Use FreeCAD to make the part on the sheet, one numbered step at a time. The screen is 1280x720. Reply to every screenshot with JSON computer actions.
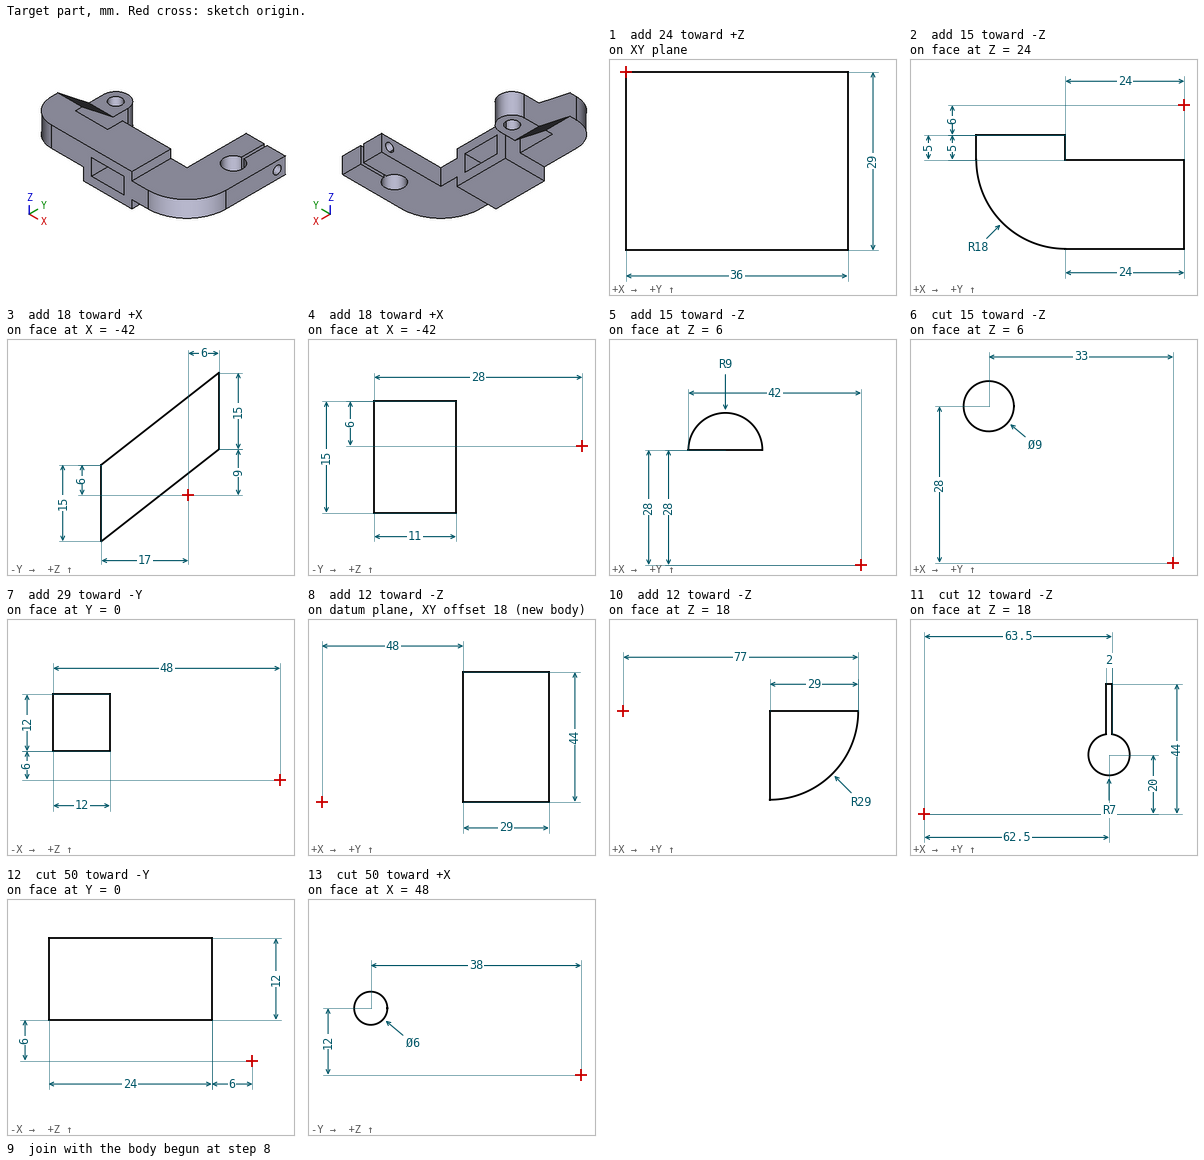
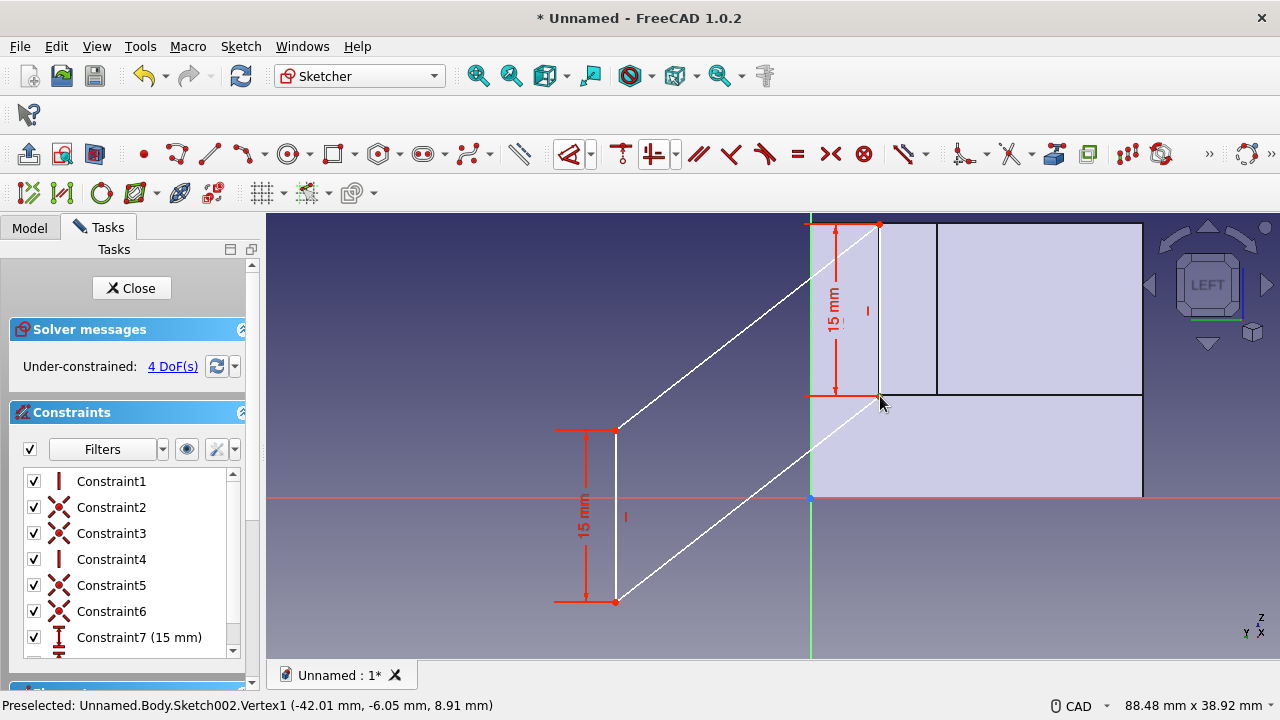
{"action": "key", "text": "l"}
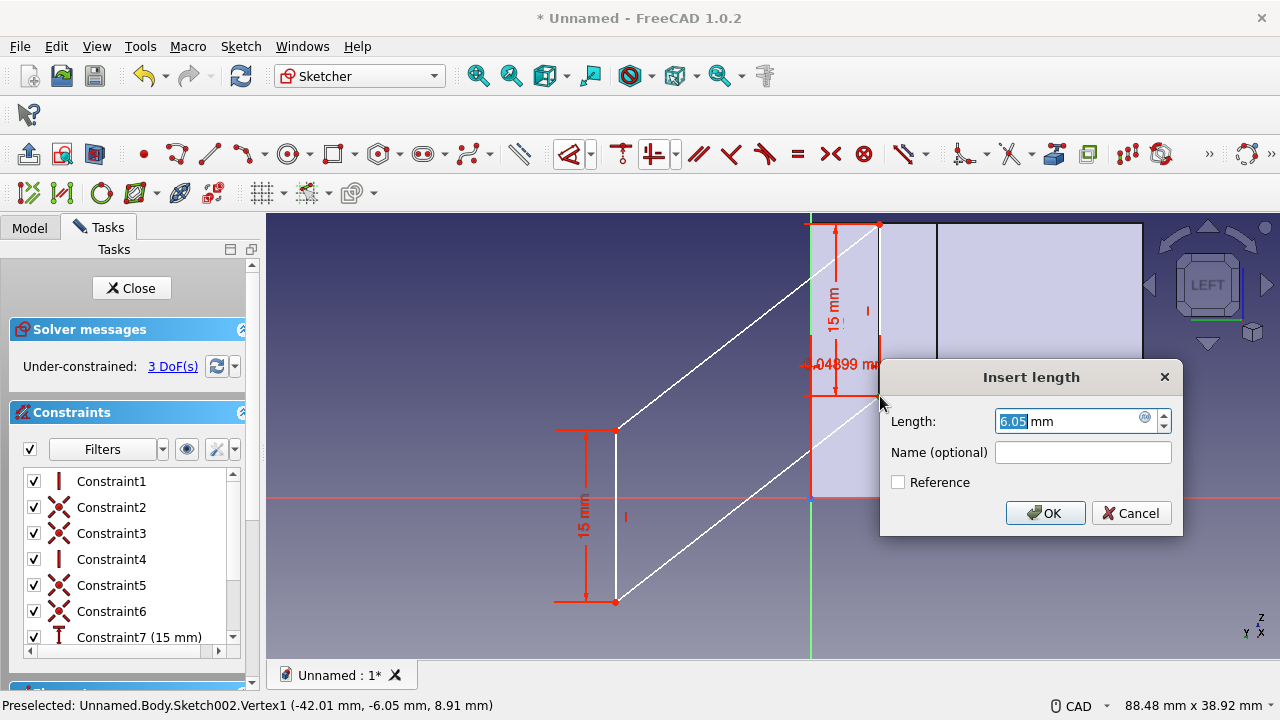
{"action": "type", "text": "6"}
{"action": "key", "text": "Return"}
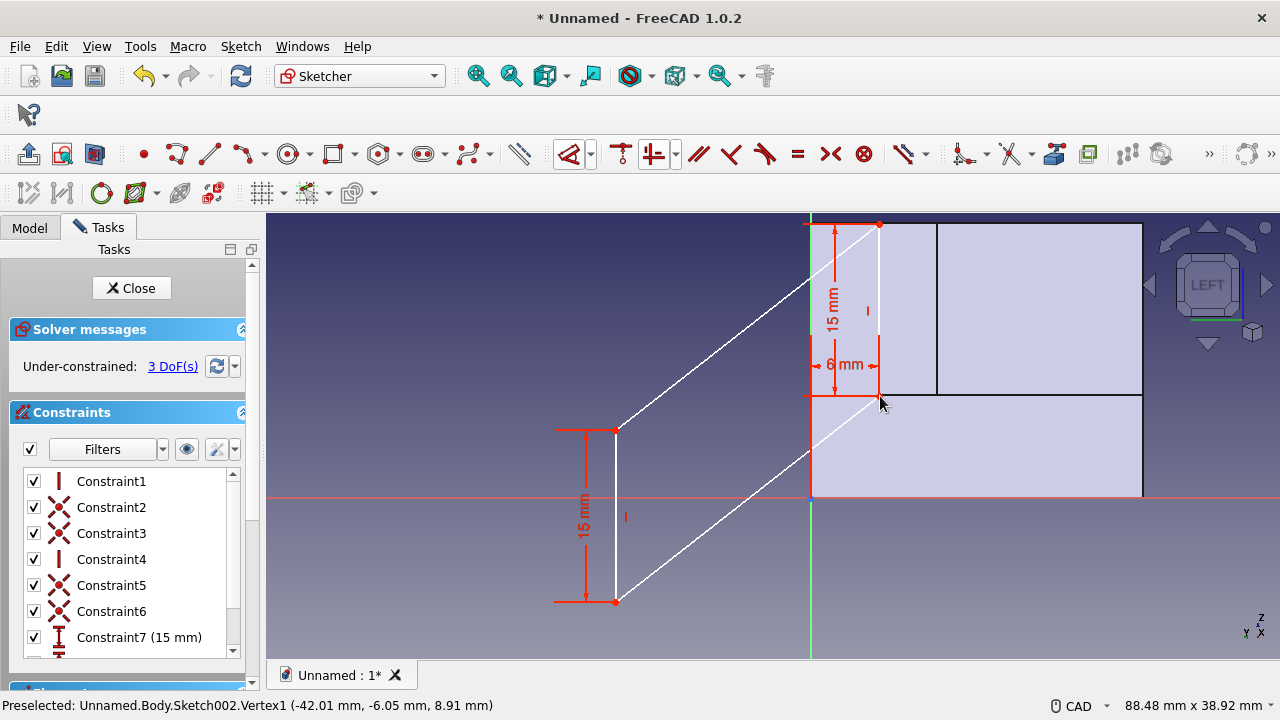
{"action": "left_click", "coordinate": [879, 396]}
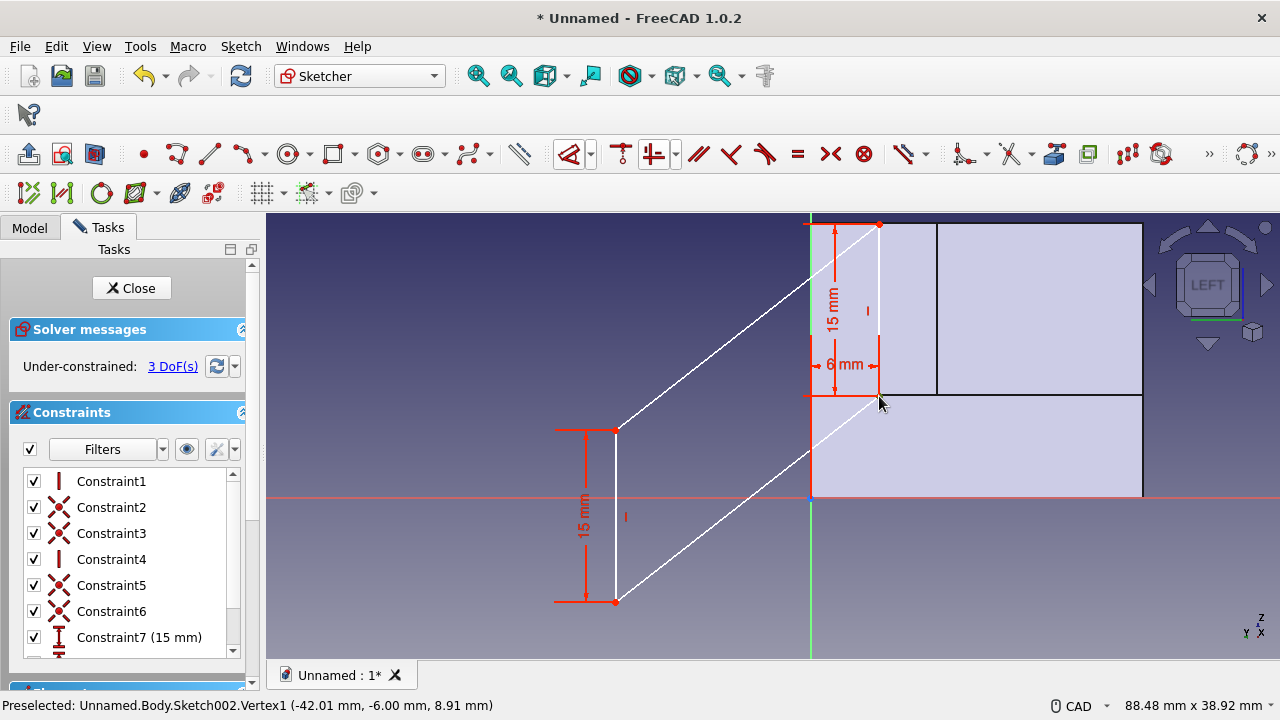
{"action": "left_click", "coordinate": [590, 154]}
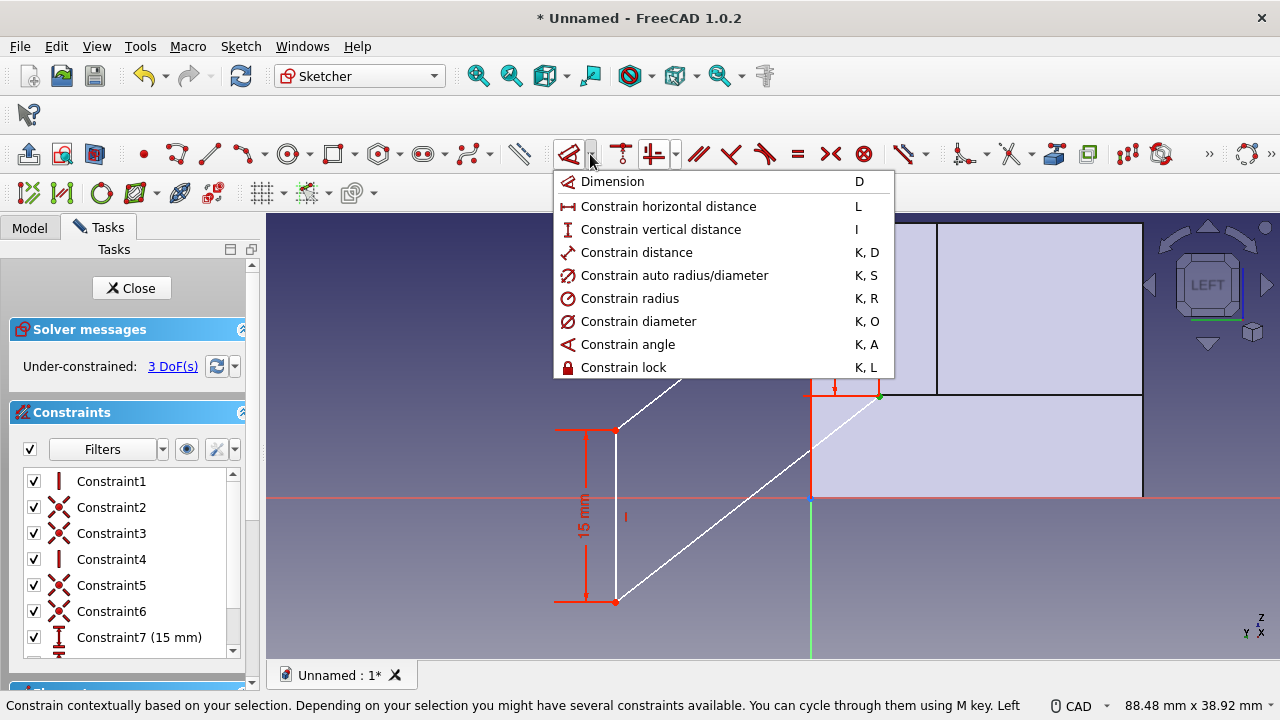
{"action": "left_click", "coordinate": [724, 230]}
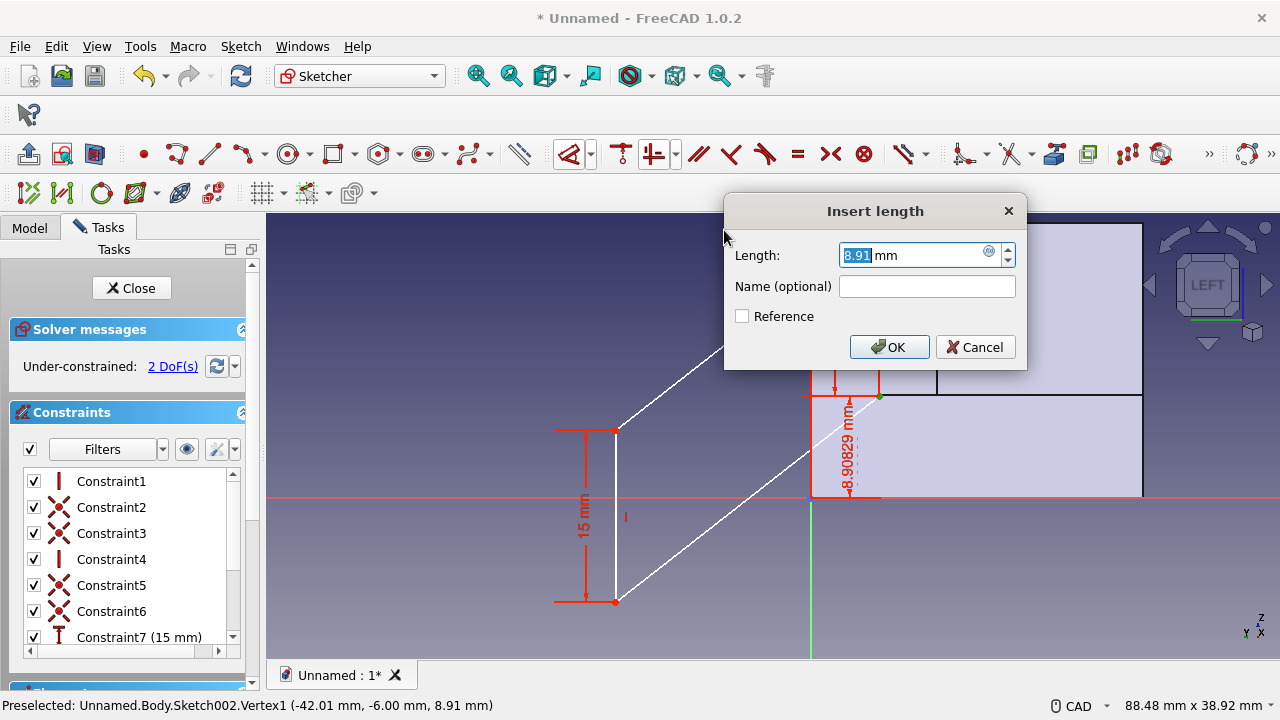
{"action": "type", "text": "9"}
{"action": "key", "text": "Return"}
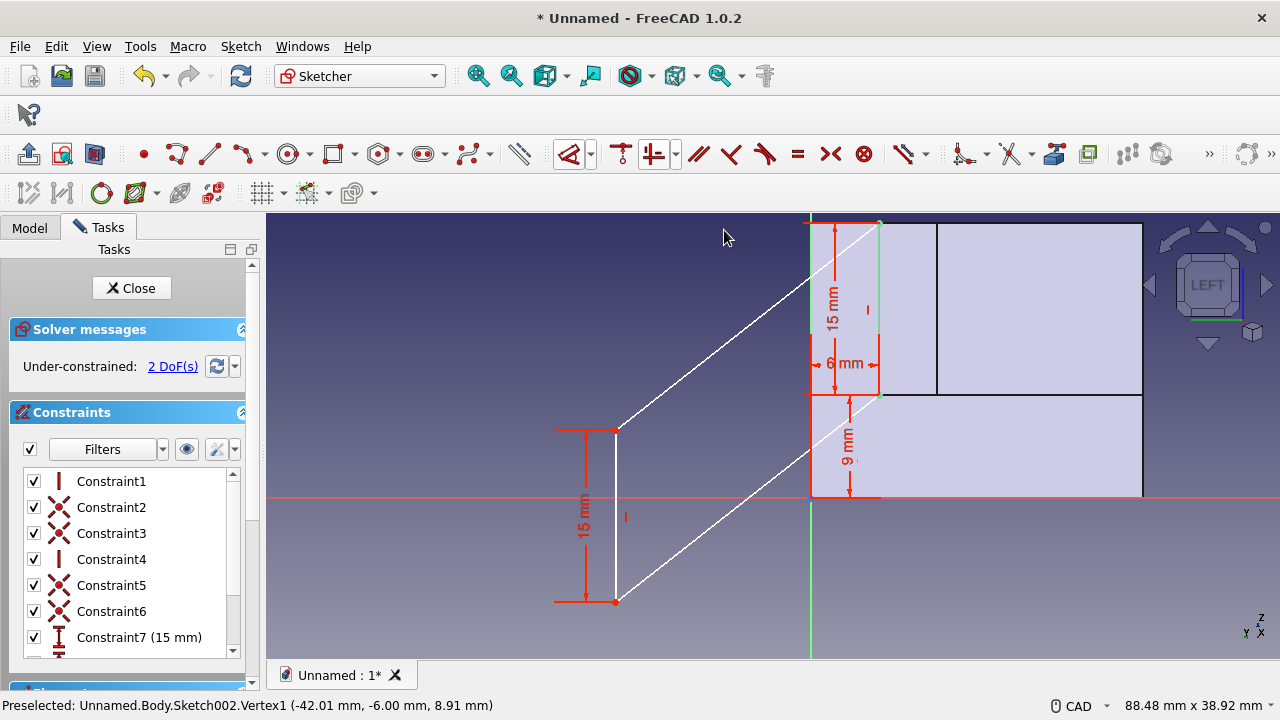
{"action": "left_click", "coordinate": [616, 430]}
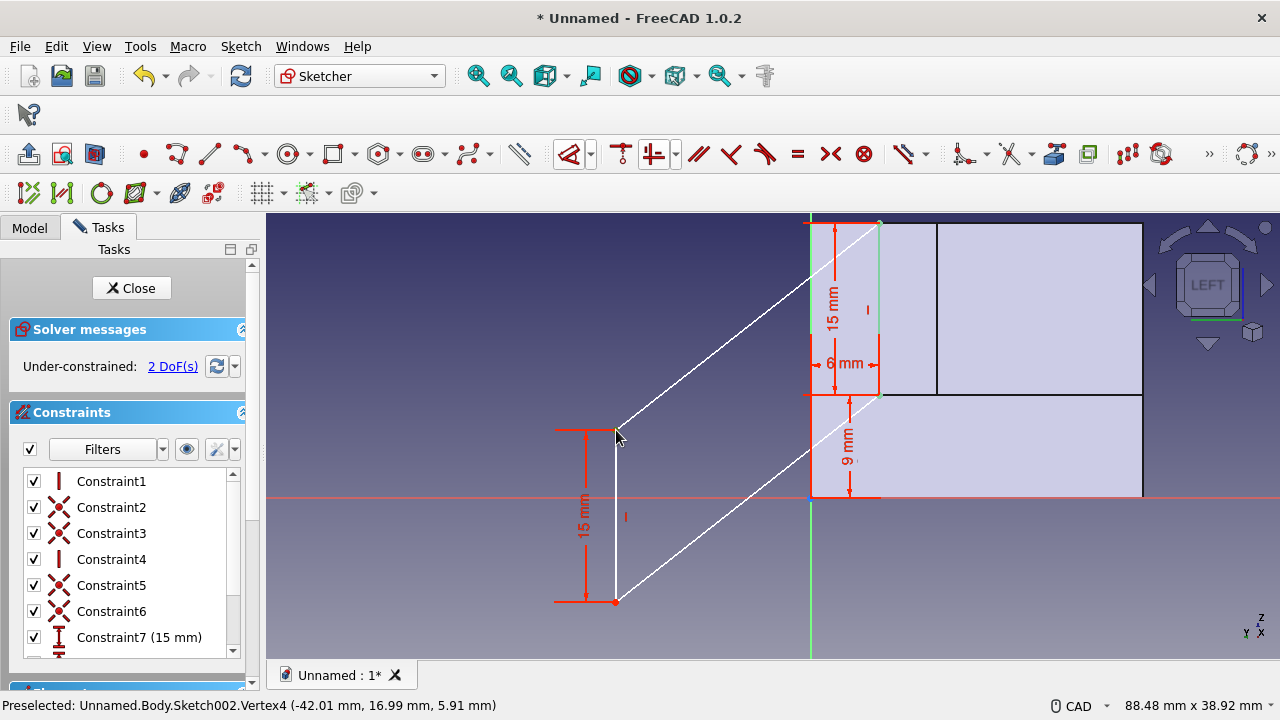
{"action": "left_click", "coordinate": [590, 154]}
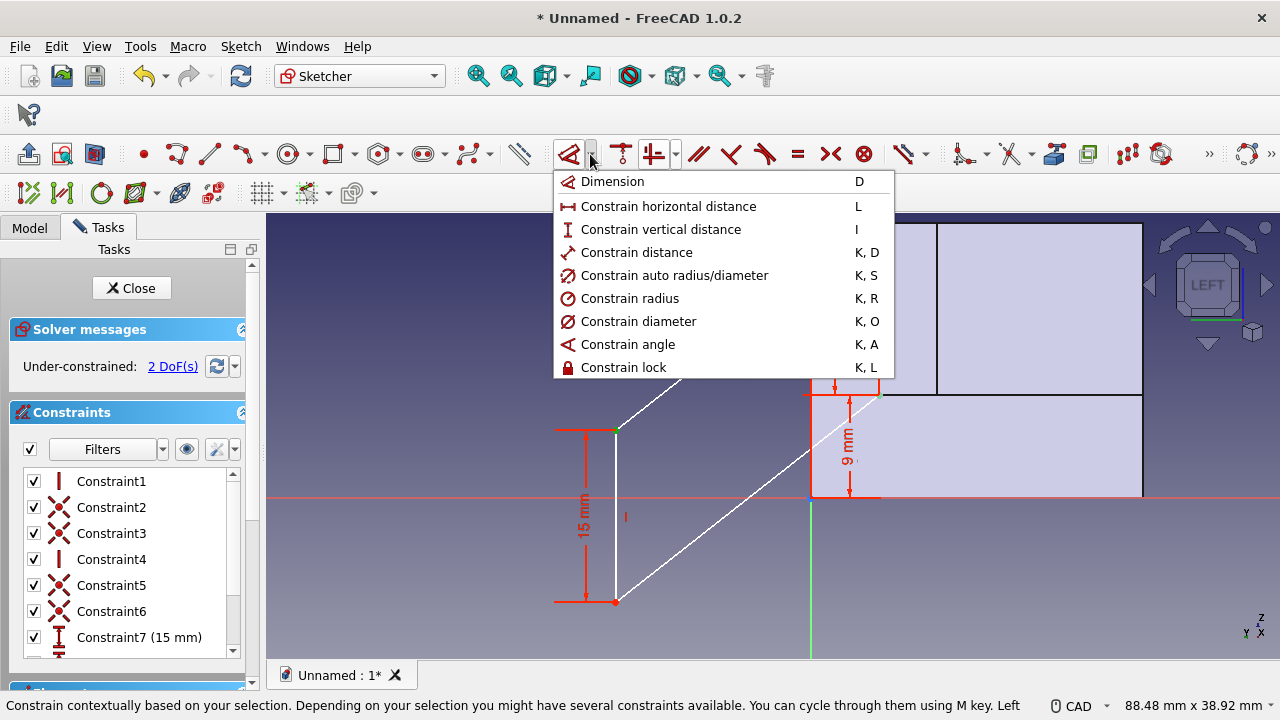
{"action": "left_click", "coordinate": [724, 230]}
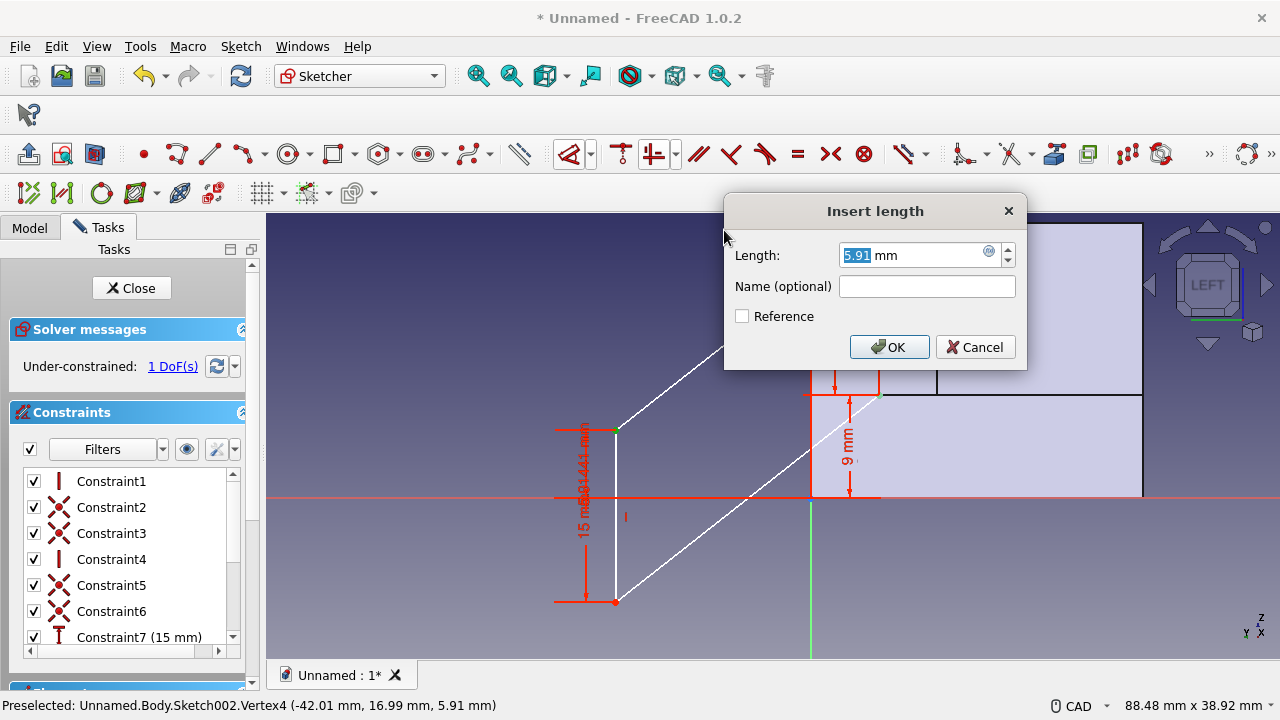
{"action": "type", "text": "6"}
{"action": "key", "text": "Return"}